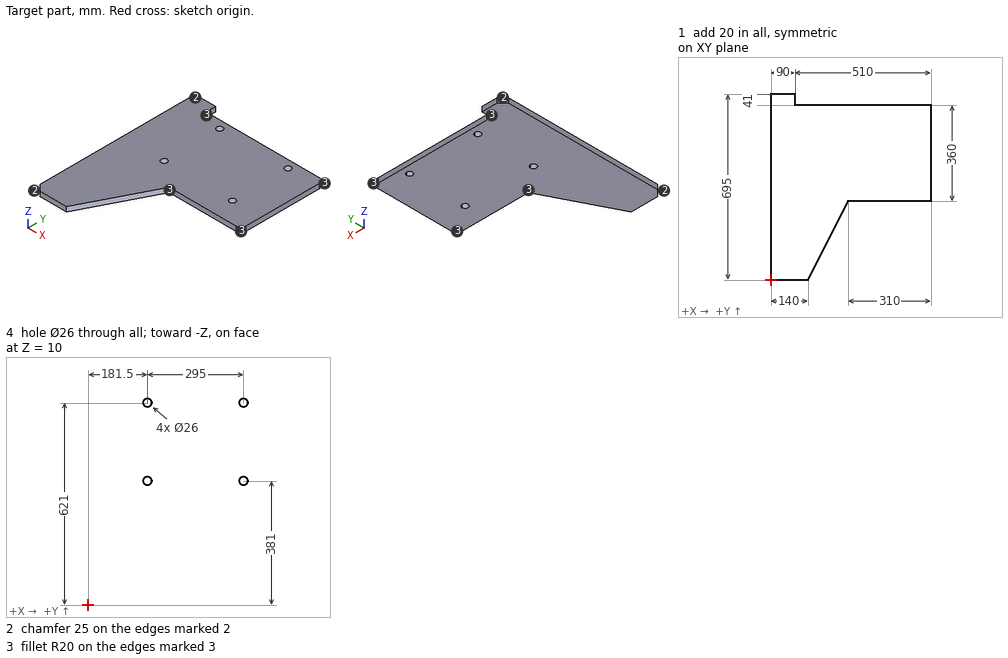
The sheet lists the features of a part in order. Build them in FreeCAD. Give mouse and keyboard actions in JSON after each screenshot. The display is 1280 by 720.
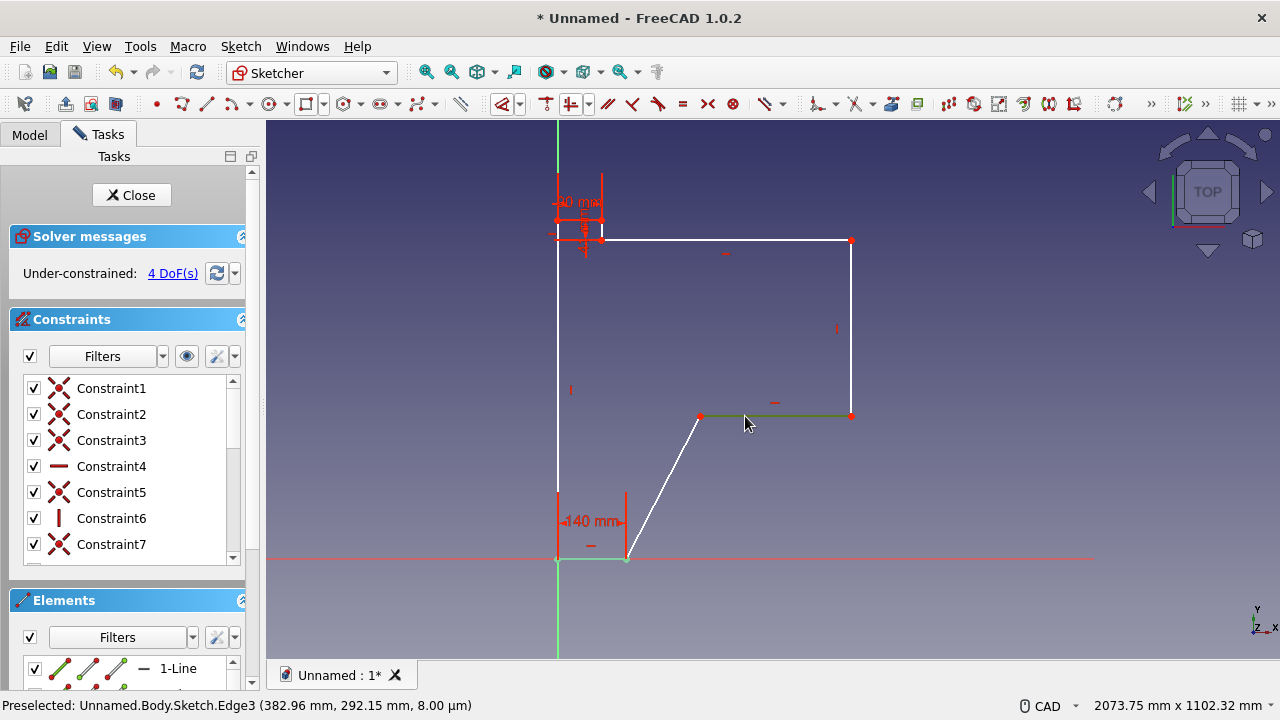
{"action": "left_click", "coordinate": [520, 104]}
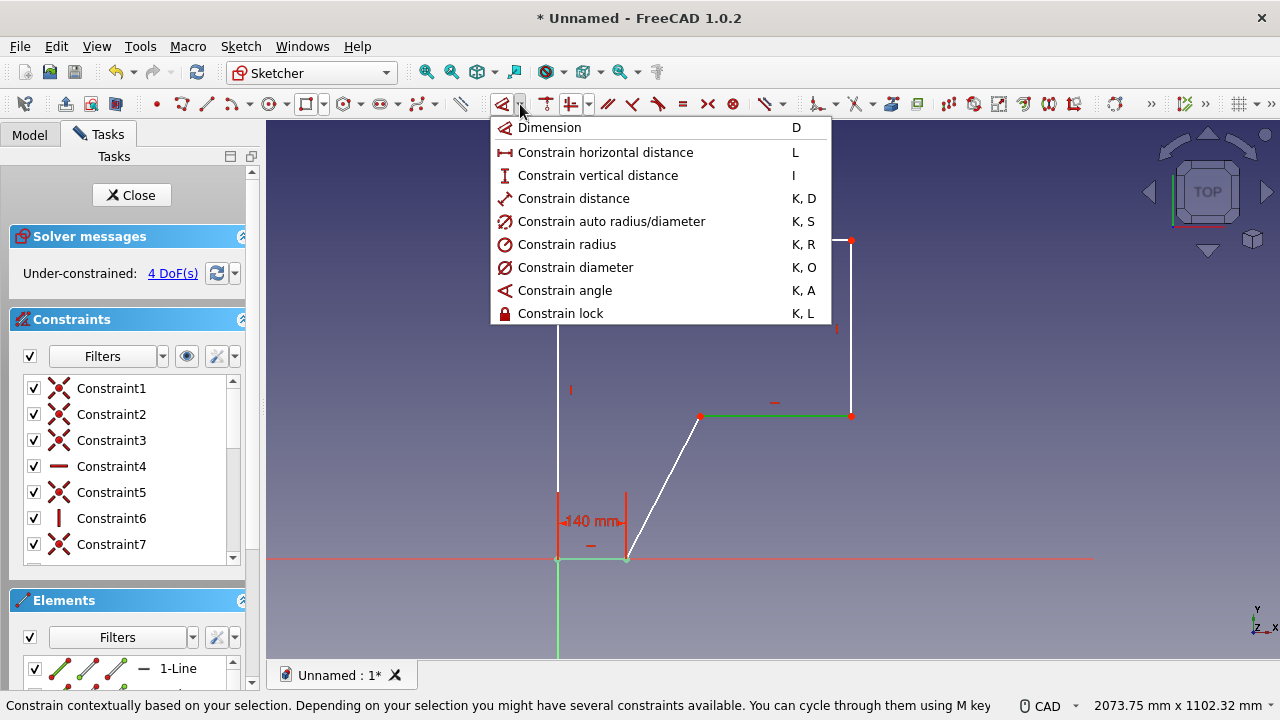
{"action": "left_click", "coordinate": [661, 152]}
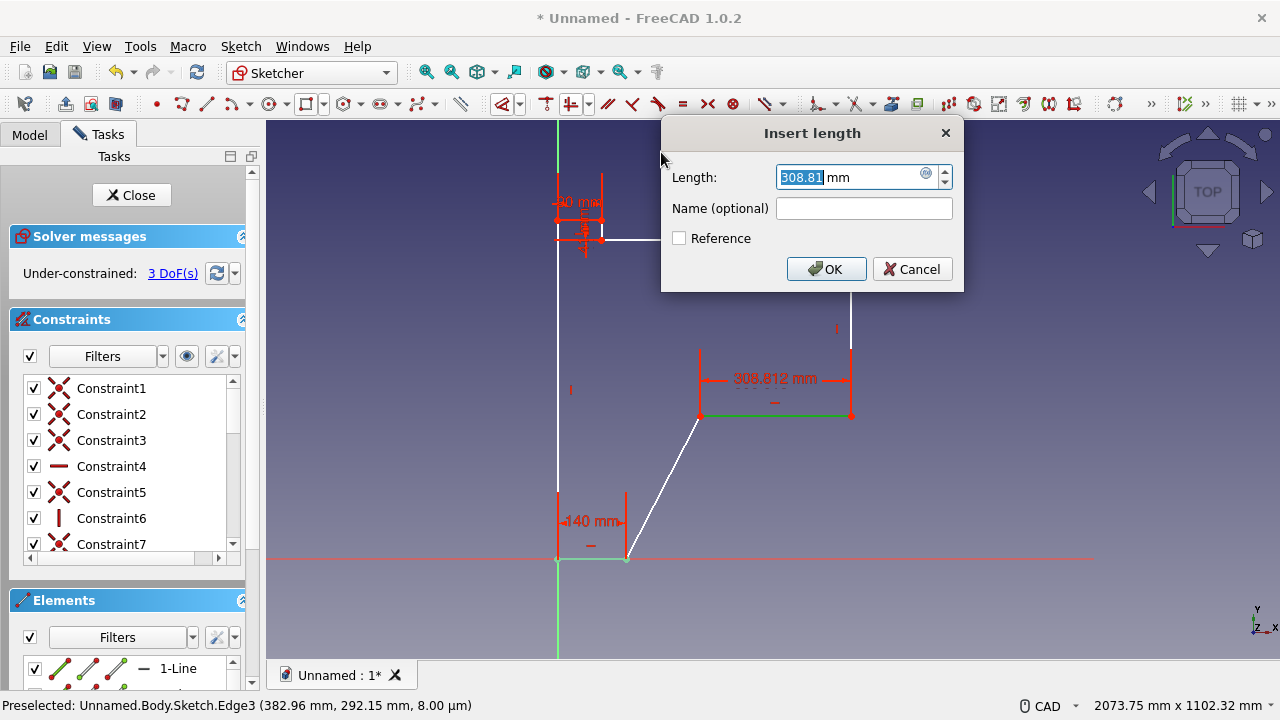
{"action": "type", "text": "310"}
{"action": "key", "text": "Return"}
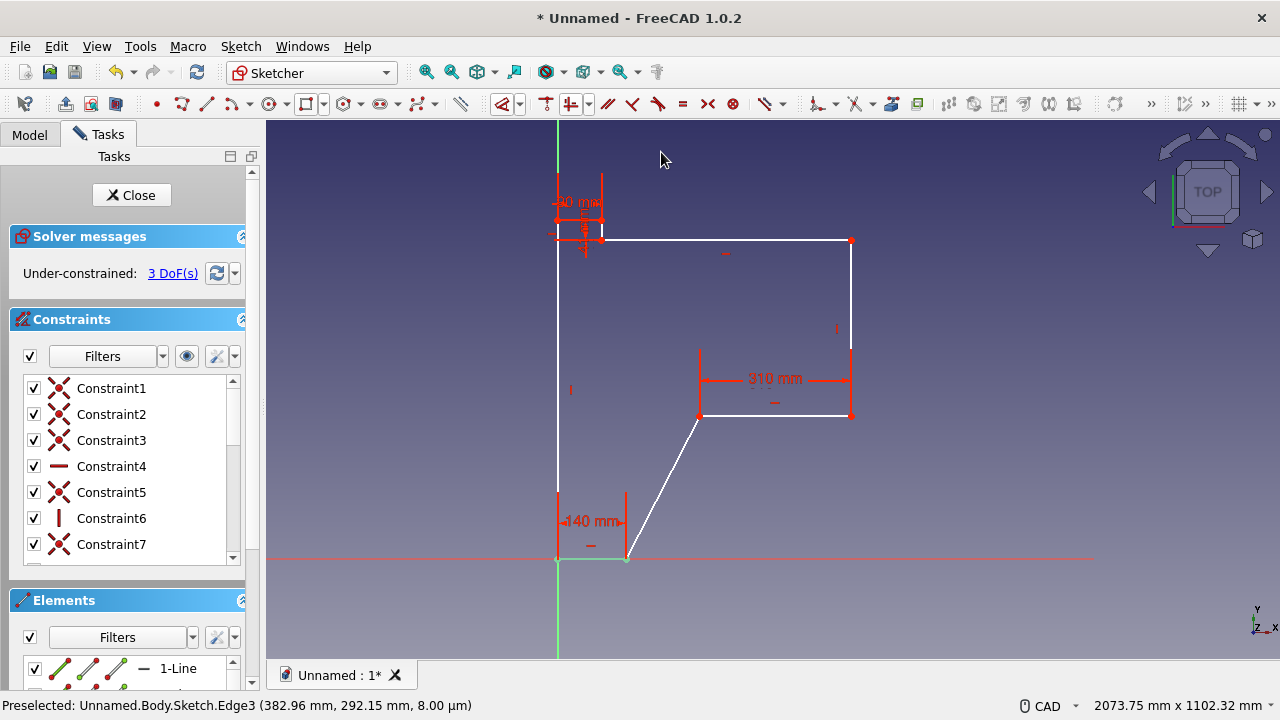
{"action": "left_click", "coordinate": [851, 364]}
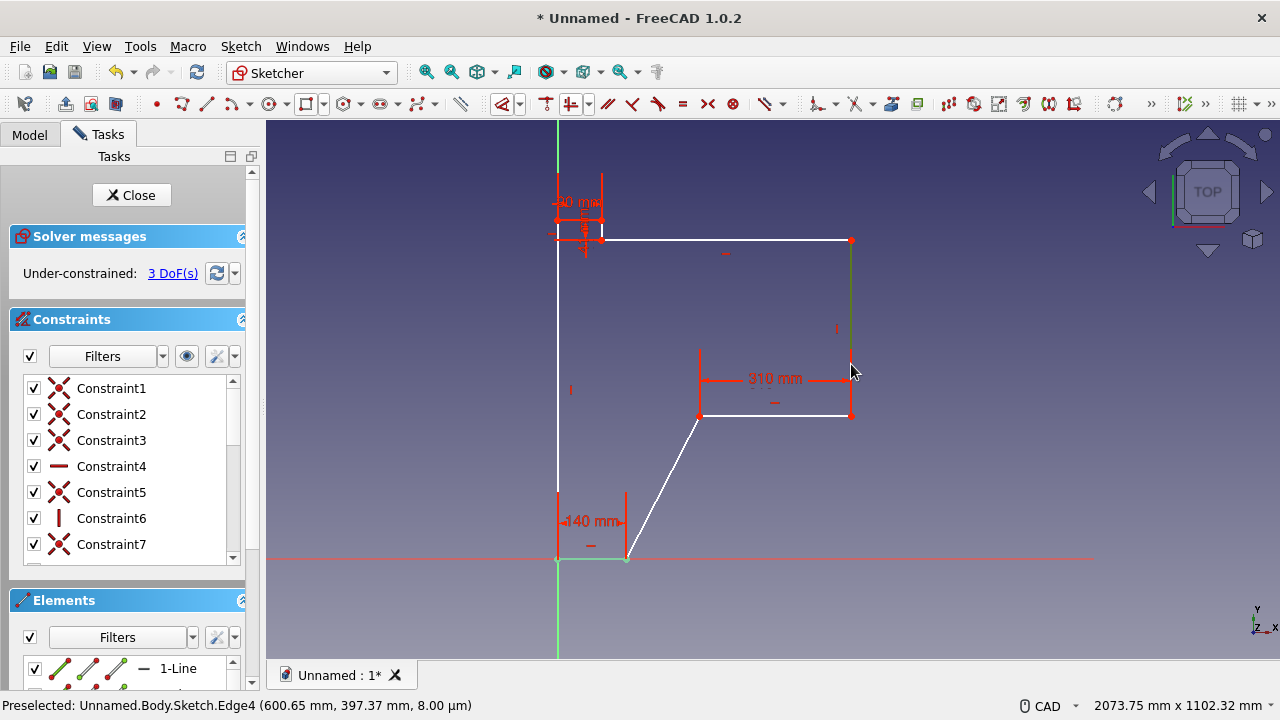
{"action": "left_click", "coordinate": [520, 104]}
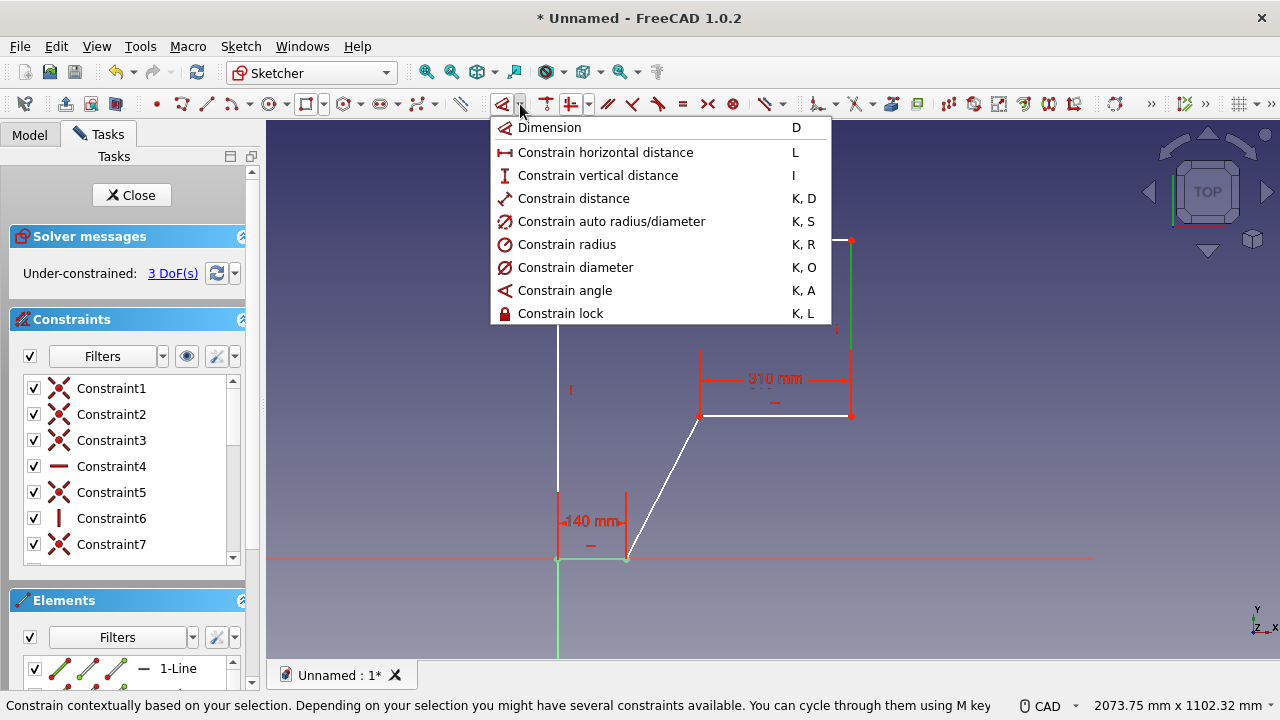
{"action": "left_click", "coordinate": [661, 176]}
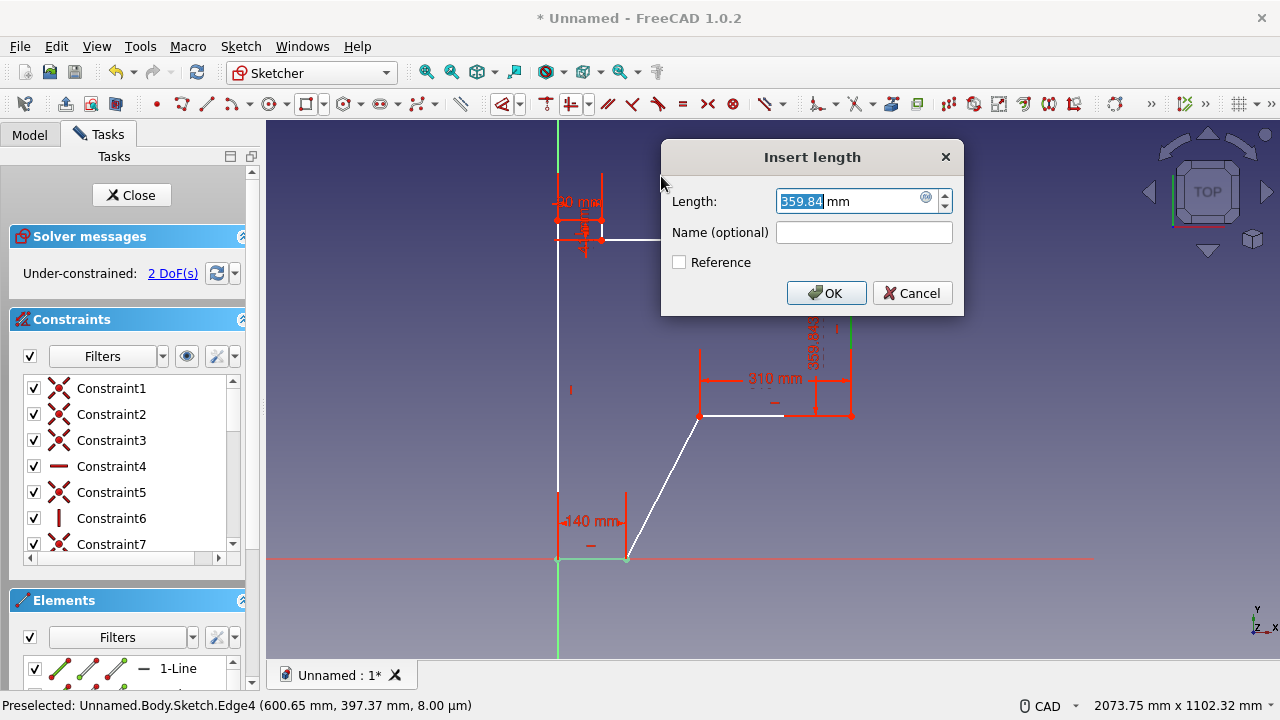
{"action": "type", "text": "360"}
{"action": "key", "text": "Return"}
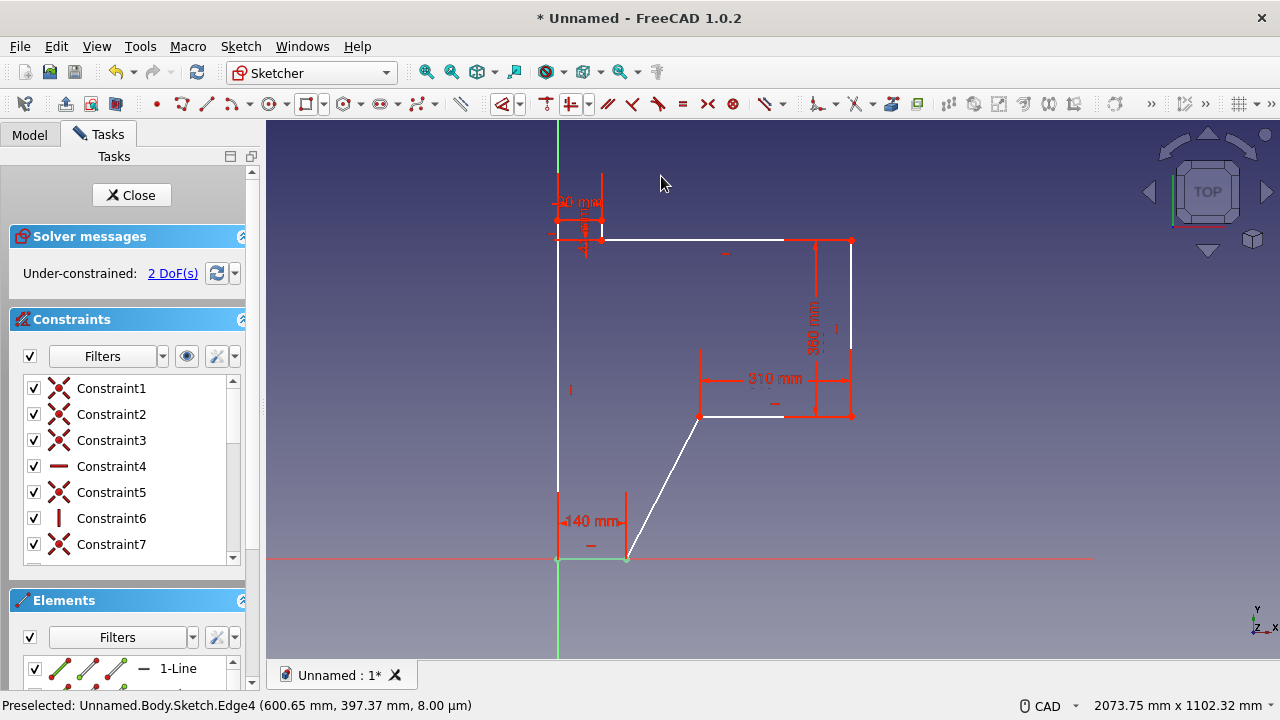
{"action": "left_click", "coordinate": [777, 240]}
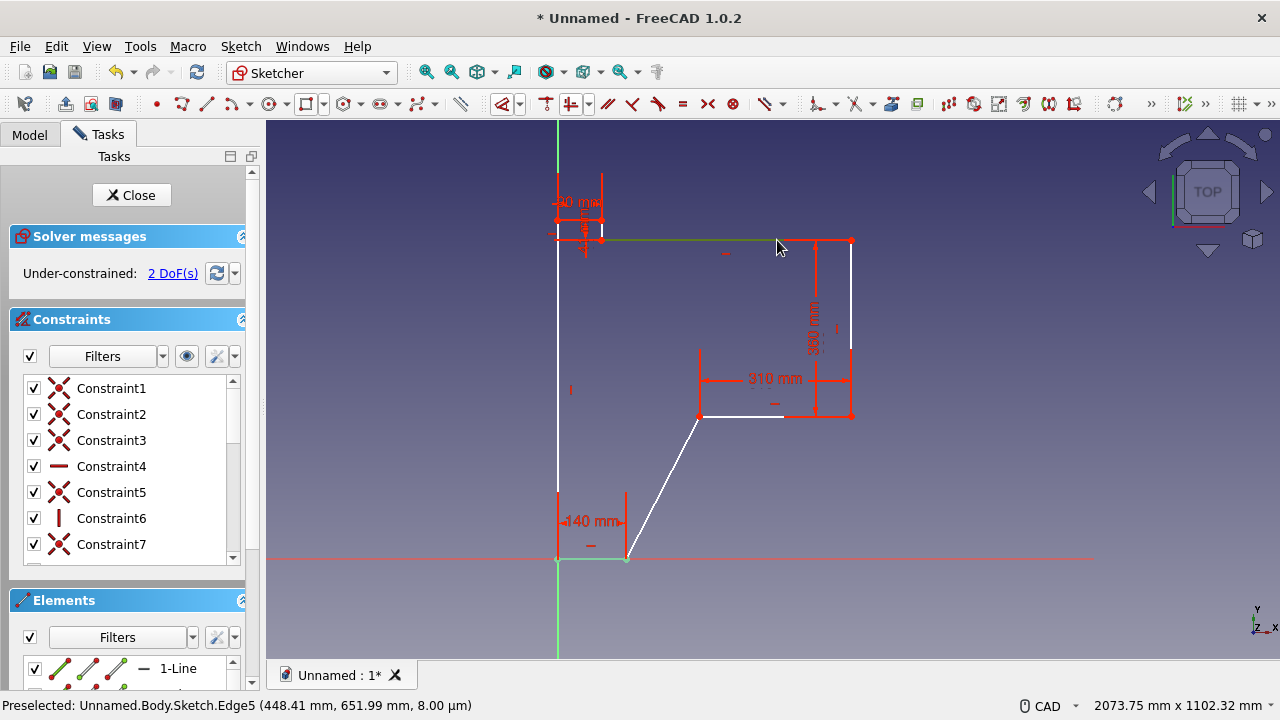
{"action": "left_click", "coordinate": [520, 104]}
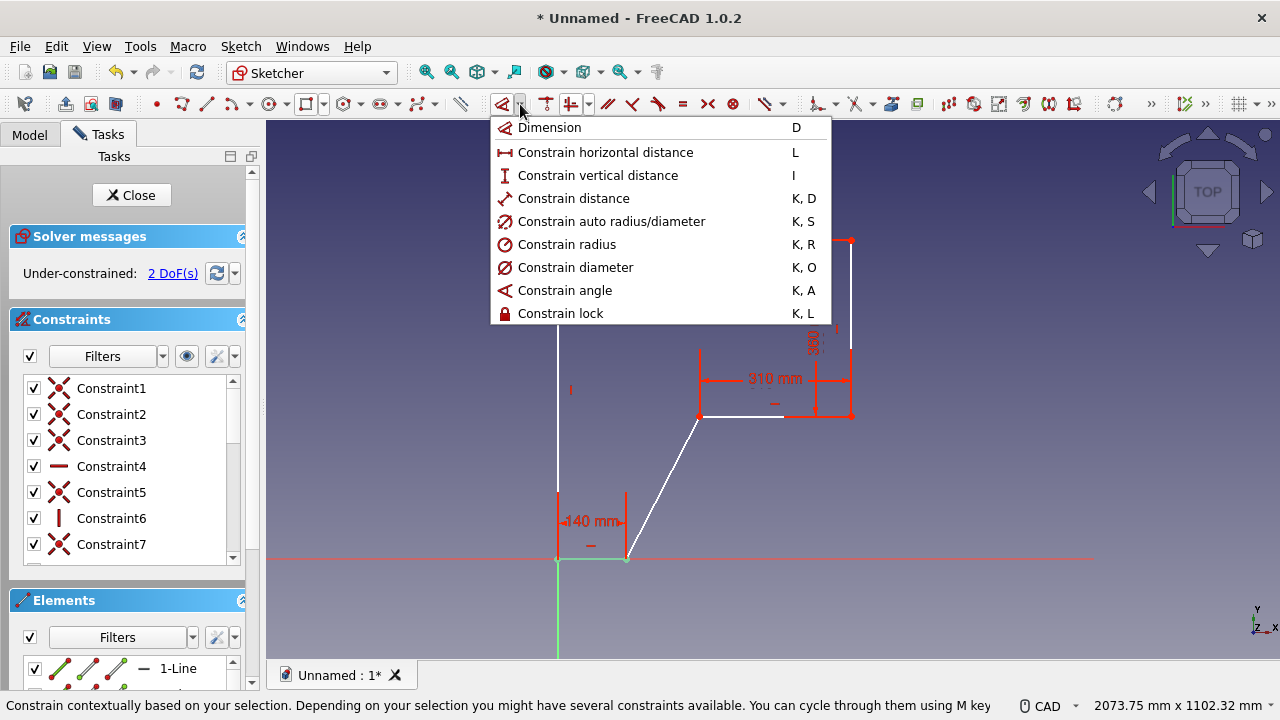
{"action": "left_click", "coordinate": [661, 152]}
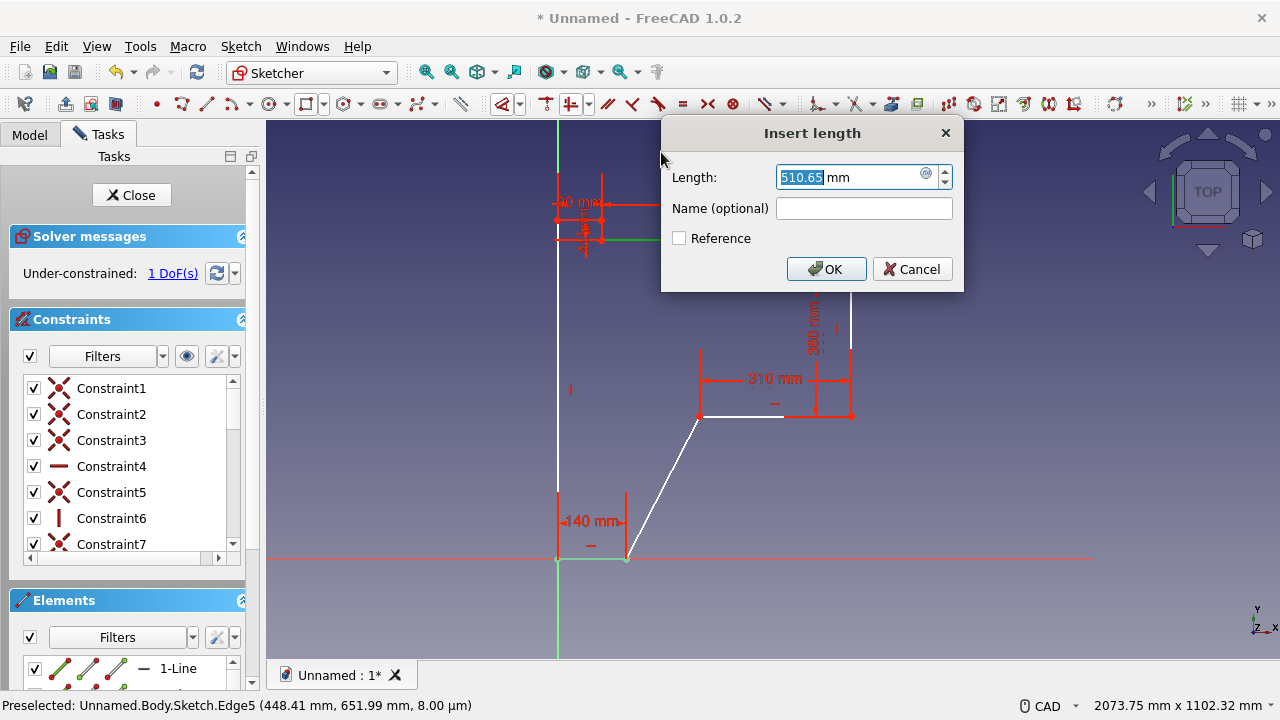
{"action": "type", "text": "510"}
{"action": "key", "text": "Return"}